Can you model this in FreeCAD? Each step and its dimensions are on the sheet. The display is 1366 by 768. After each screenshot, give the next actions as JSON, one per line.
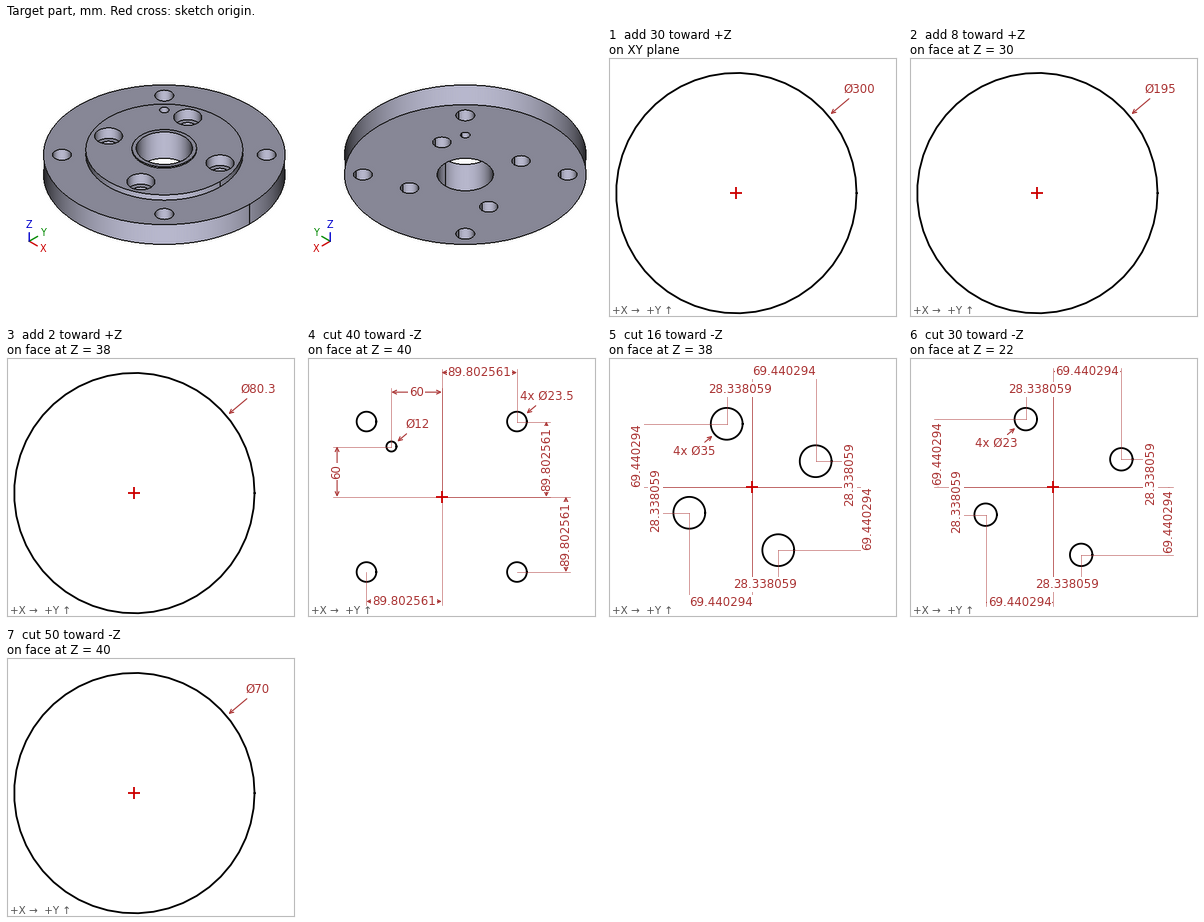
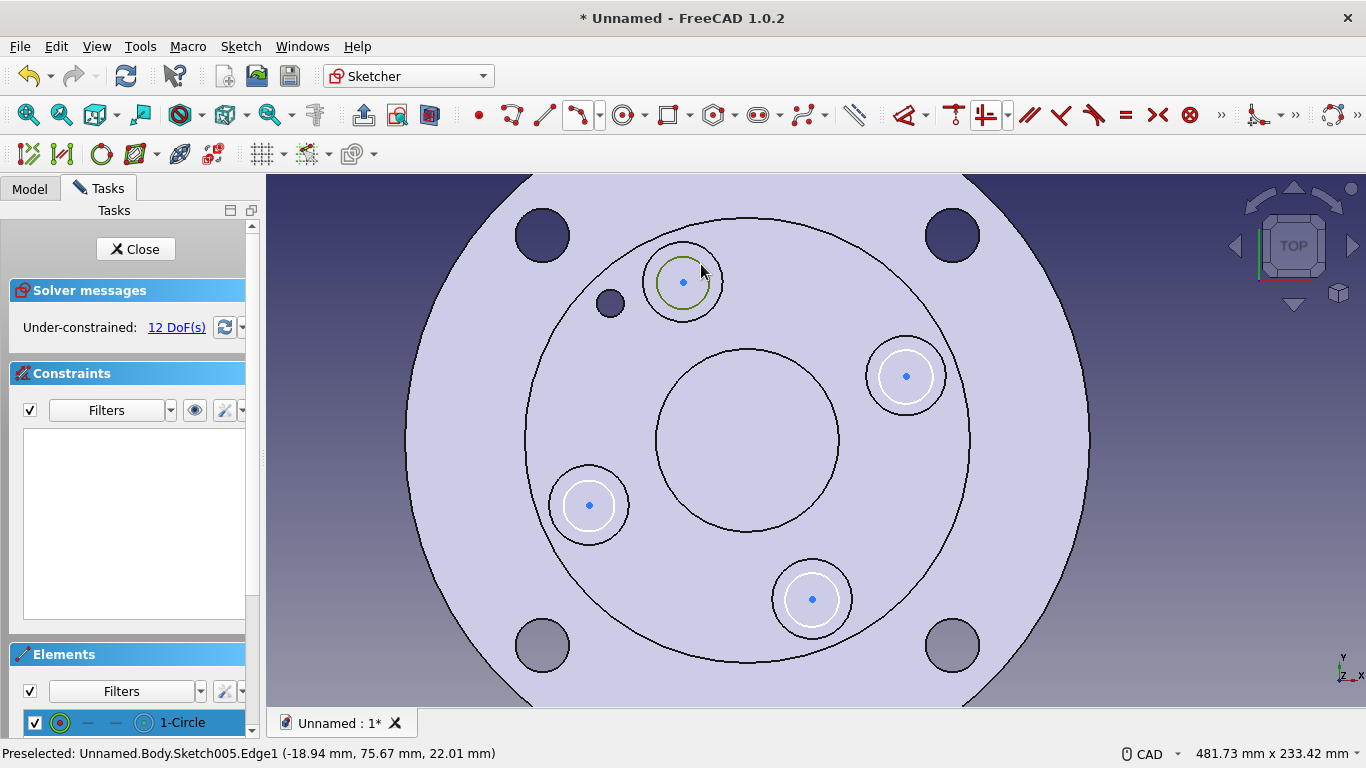
{"action": "left_click", "coordinate": [925, 358]}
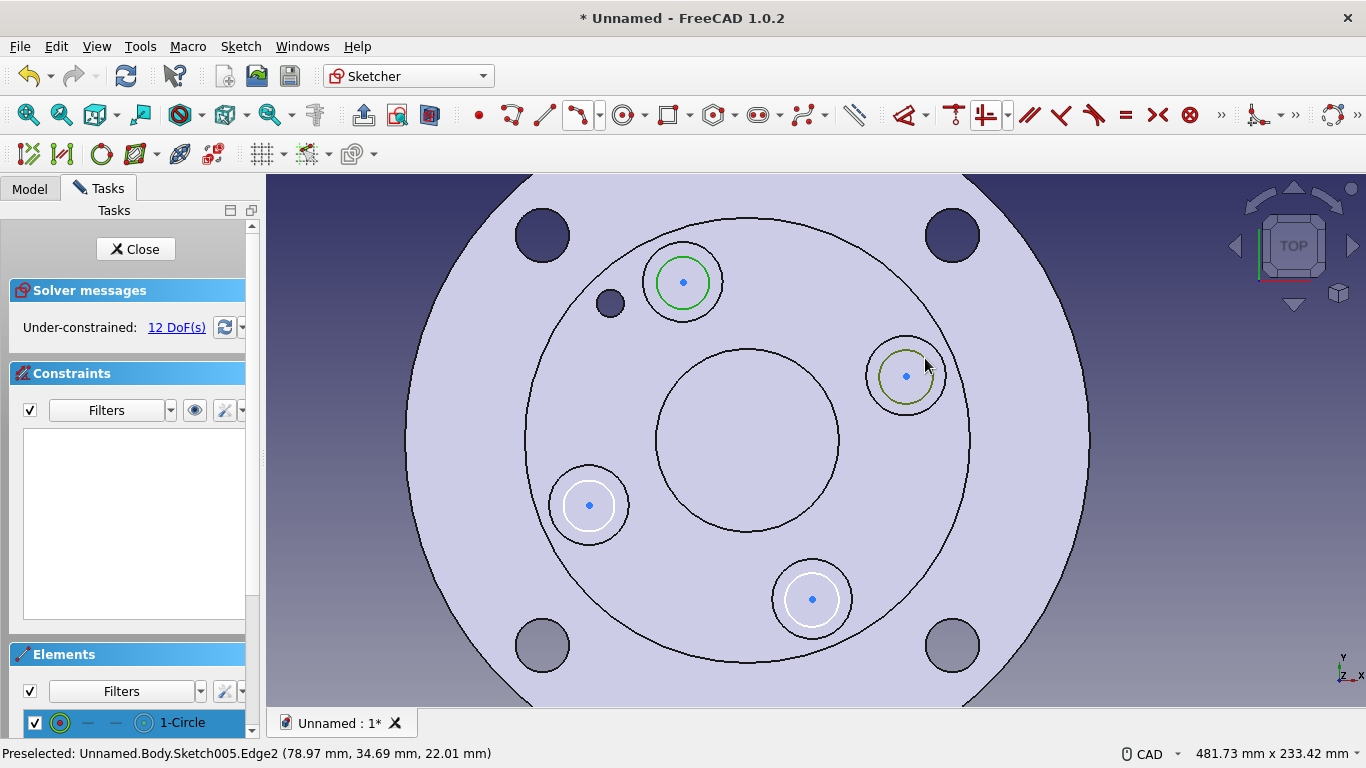
{"action": "left_click", "coordinate": [831, 581]}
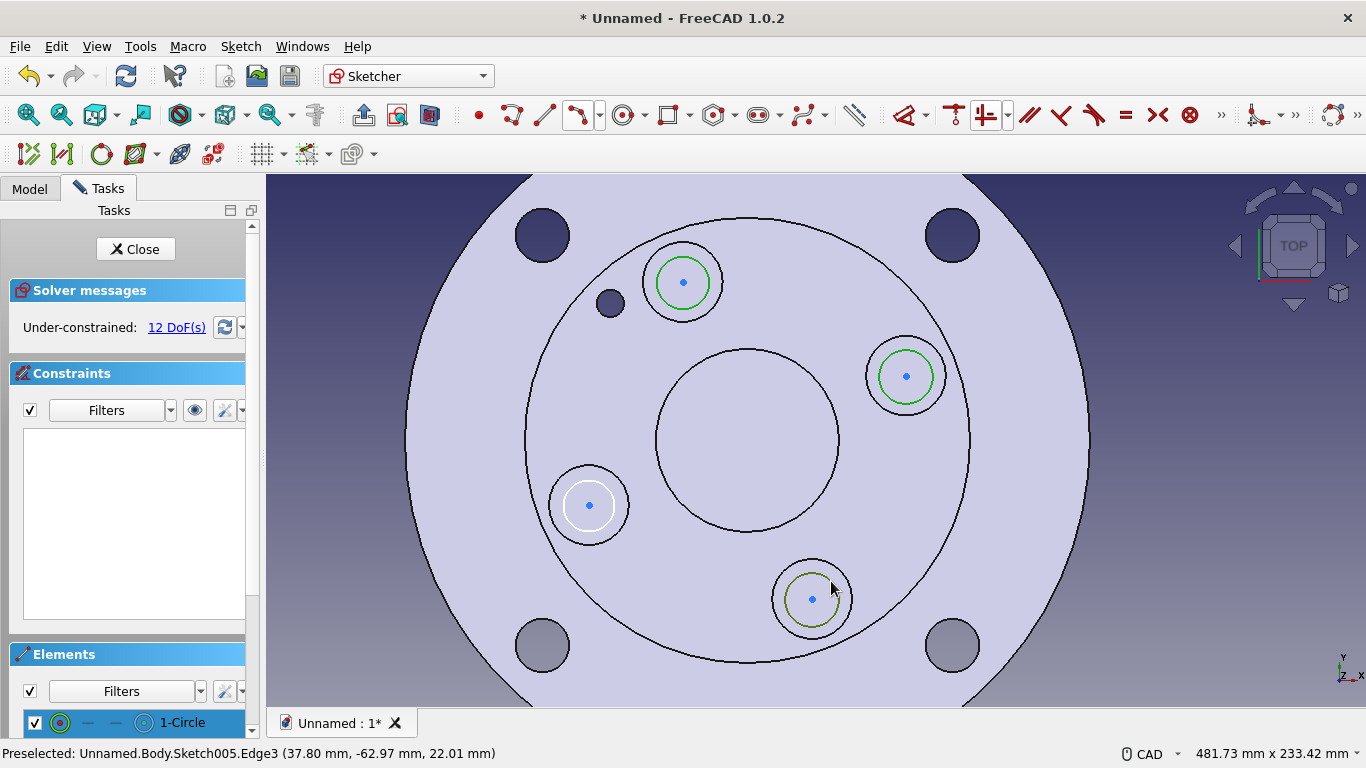
{"action": "left_click", "coordinate": [607, 488]}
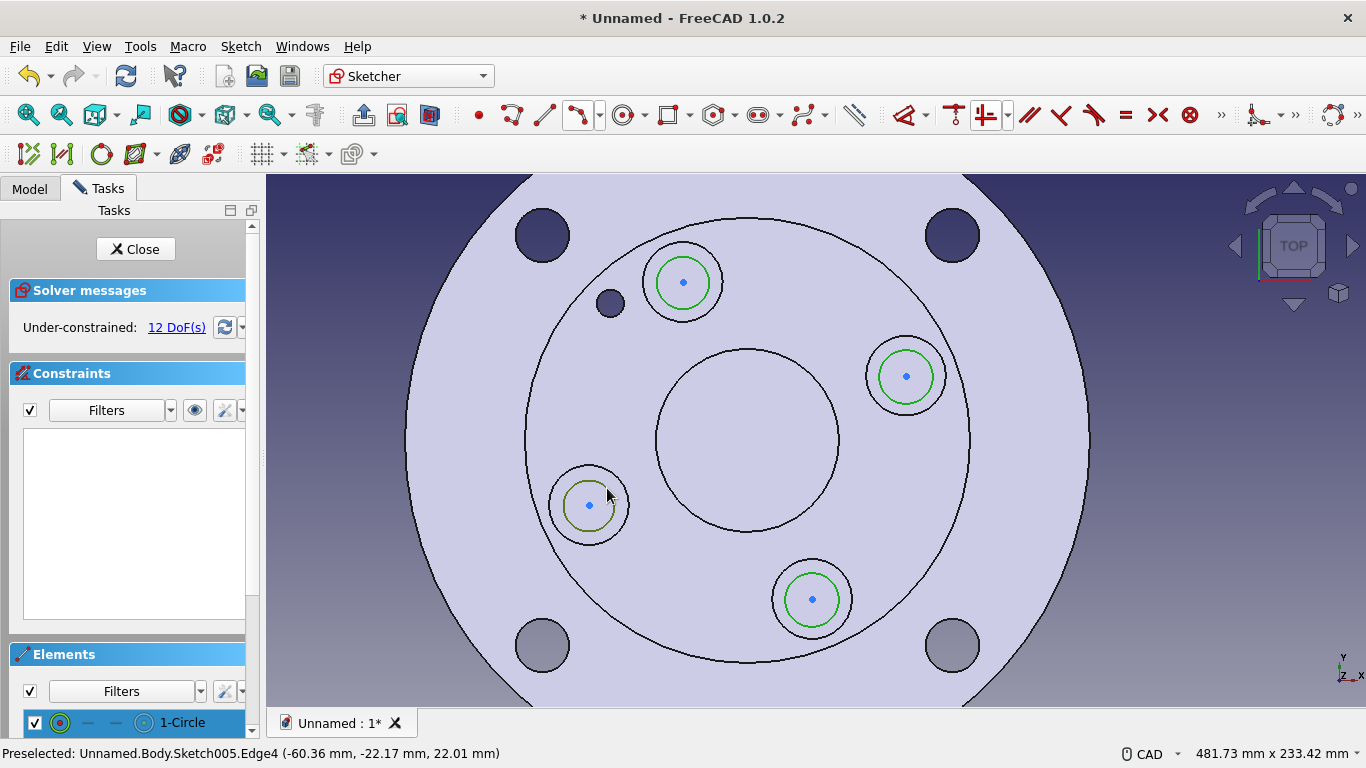
{"action": "left_click", "coordinate": [1126, 116]}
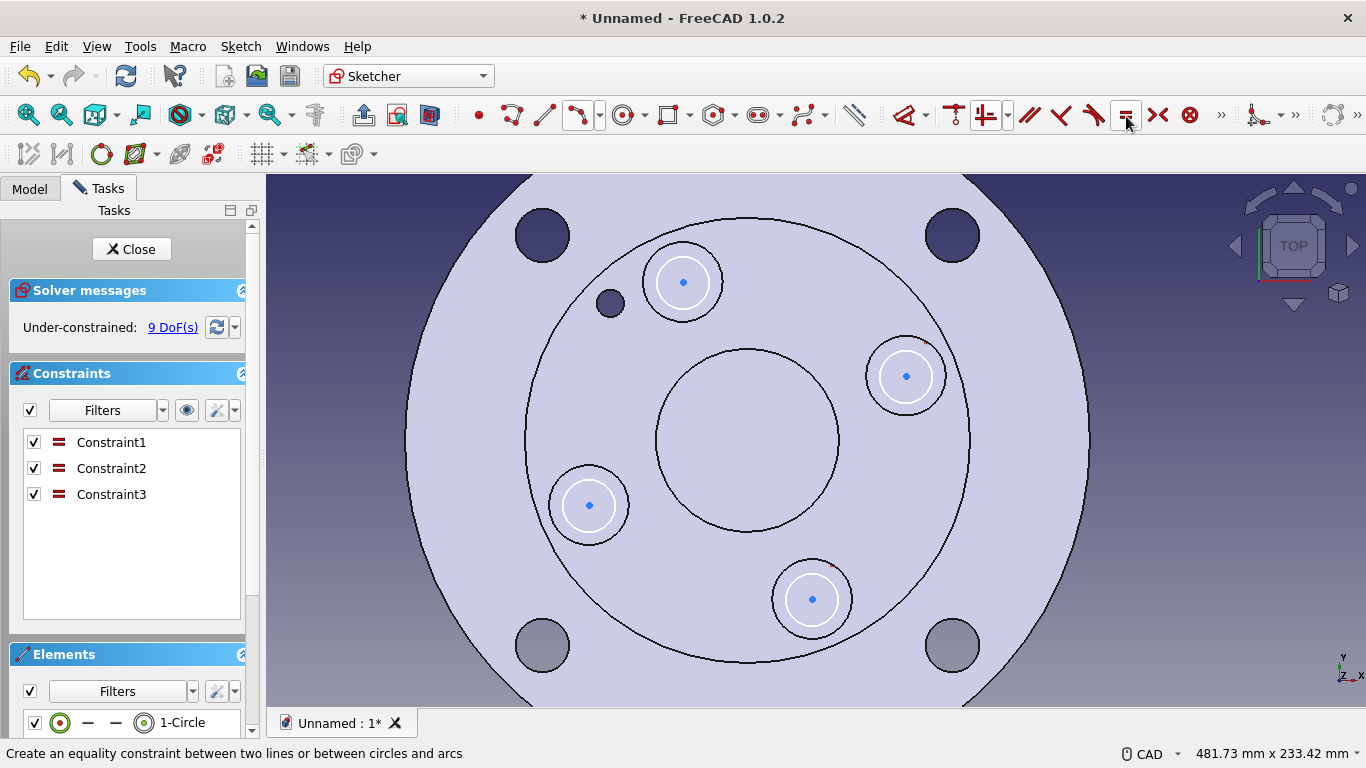
{"action": "key", "text": "d"}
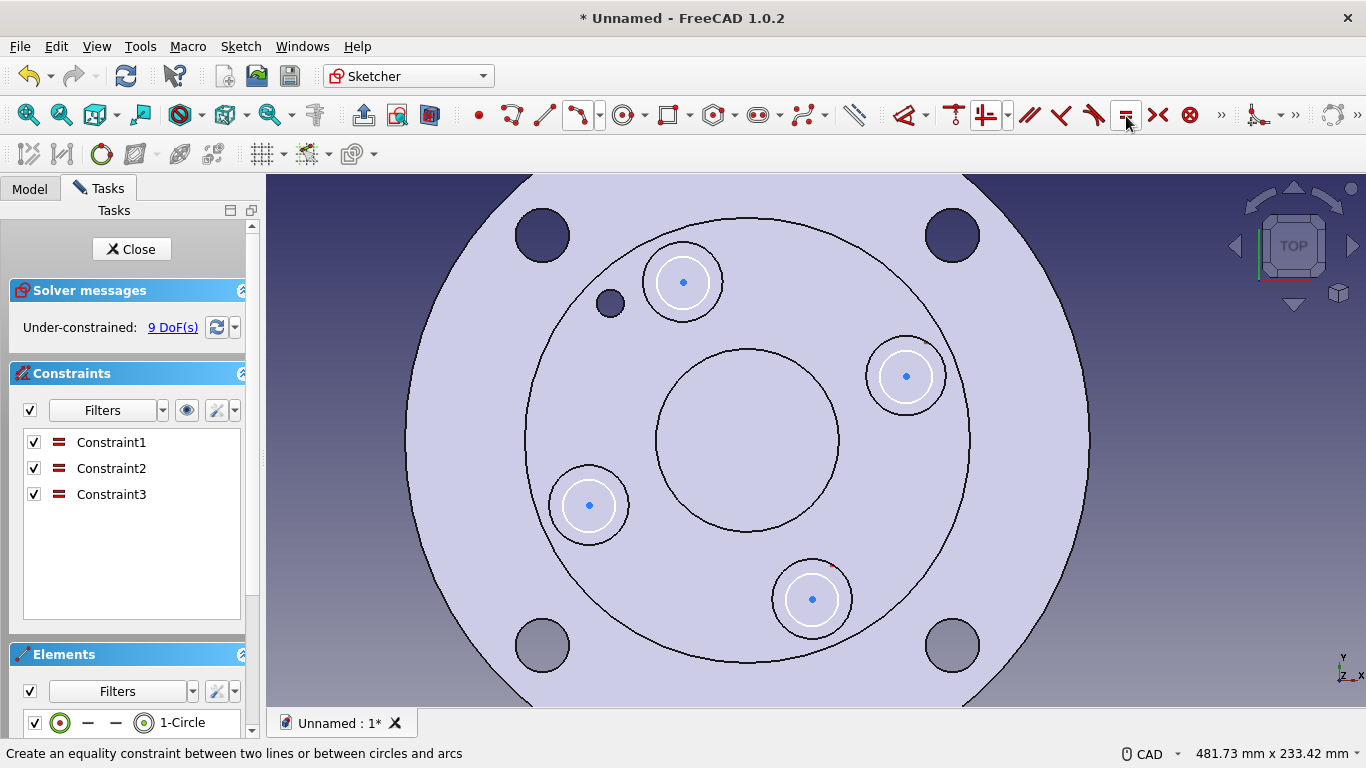
{"action": "left_click", "coordinate": [701, 264]}
{"action": "left_click", "coordinate": [723, 241]}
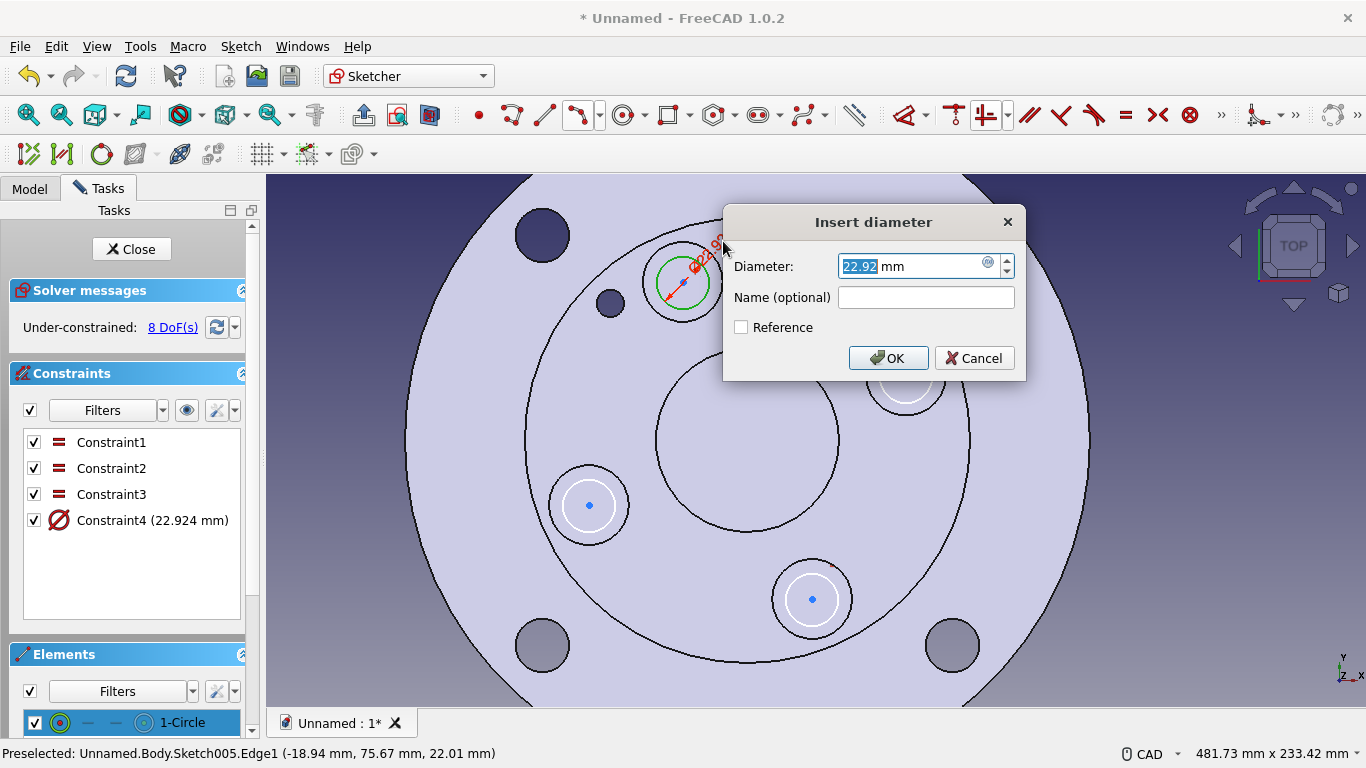
{"action": "type", "text": "23"}
{"action": "key", "text": "Return"}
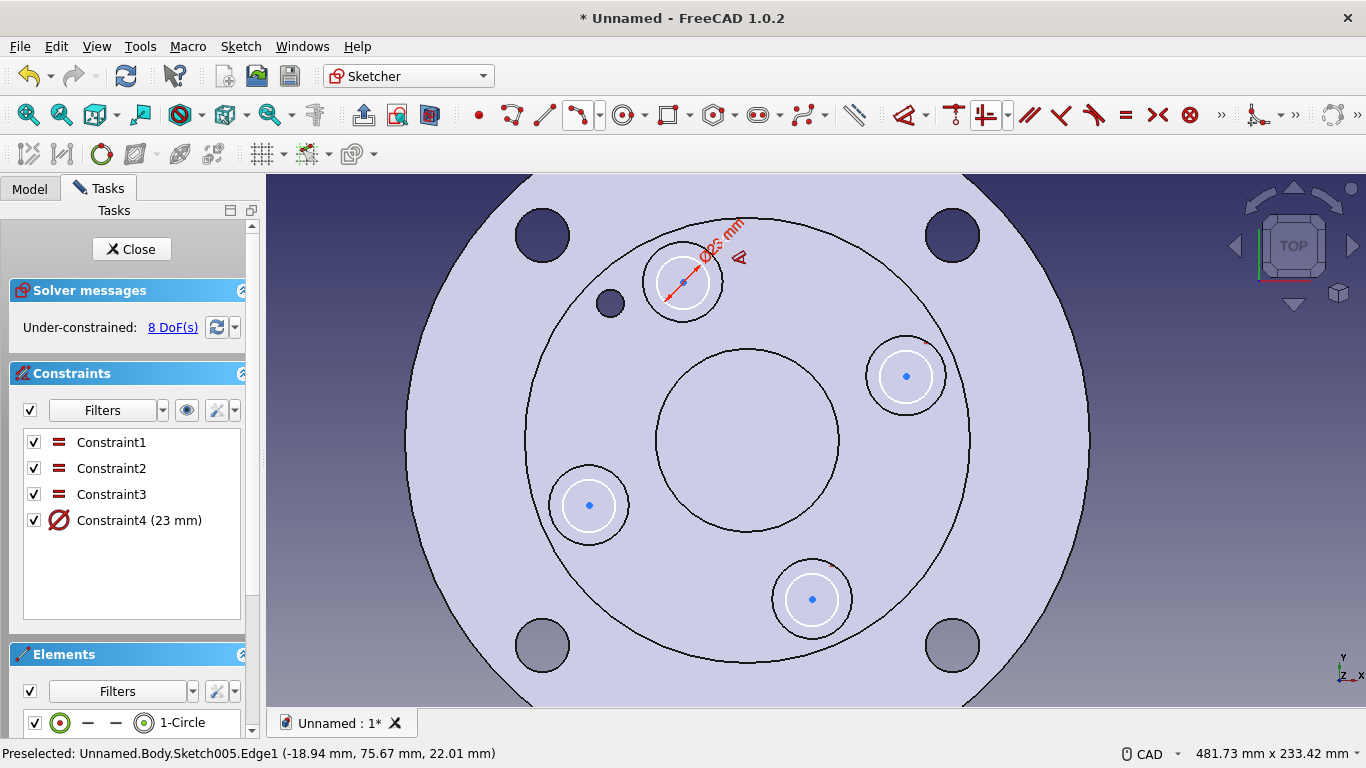
{"action": "left_click", "coordinate": [683, 283]}
{"action": "left_click", "coordinate": [715, 474]}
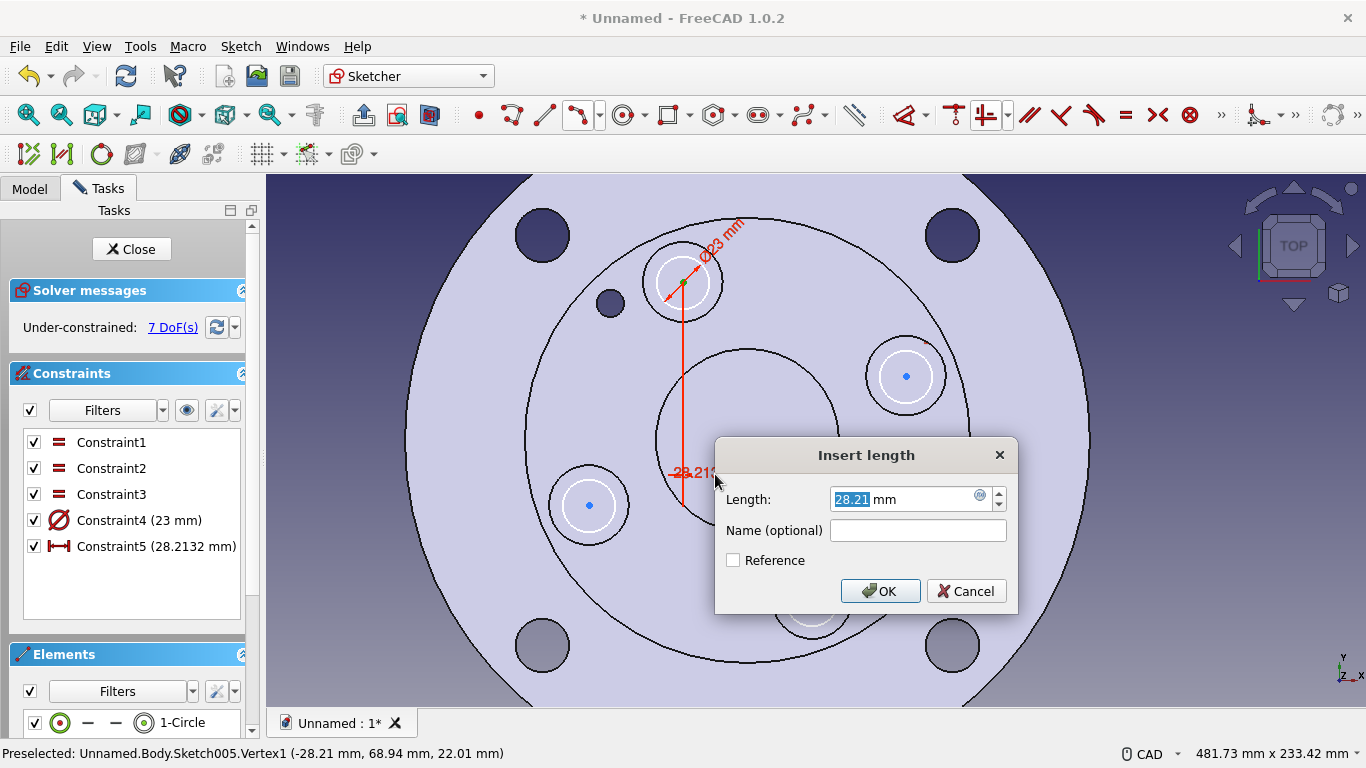
{"action": "type", "text": "28.338059"}
{"action": "key", "text": "Return"}